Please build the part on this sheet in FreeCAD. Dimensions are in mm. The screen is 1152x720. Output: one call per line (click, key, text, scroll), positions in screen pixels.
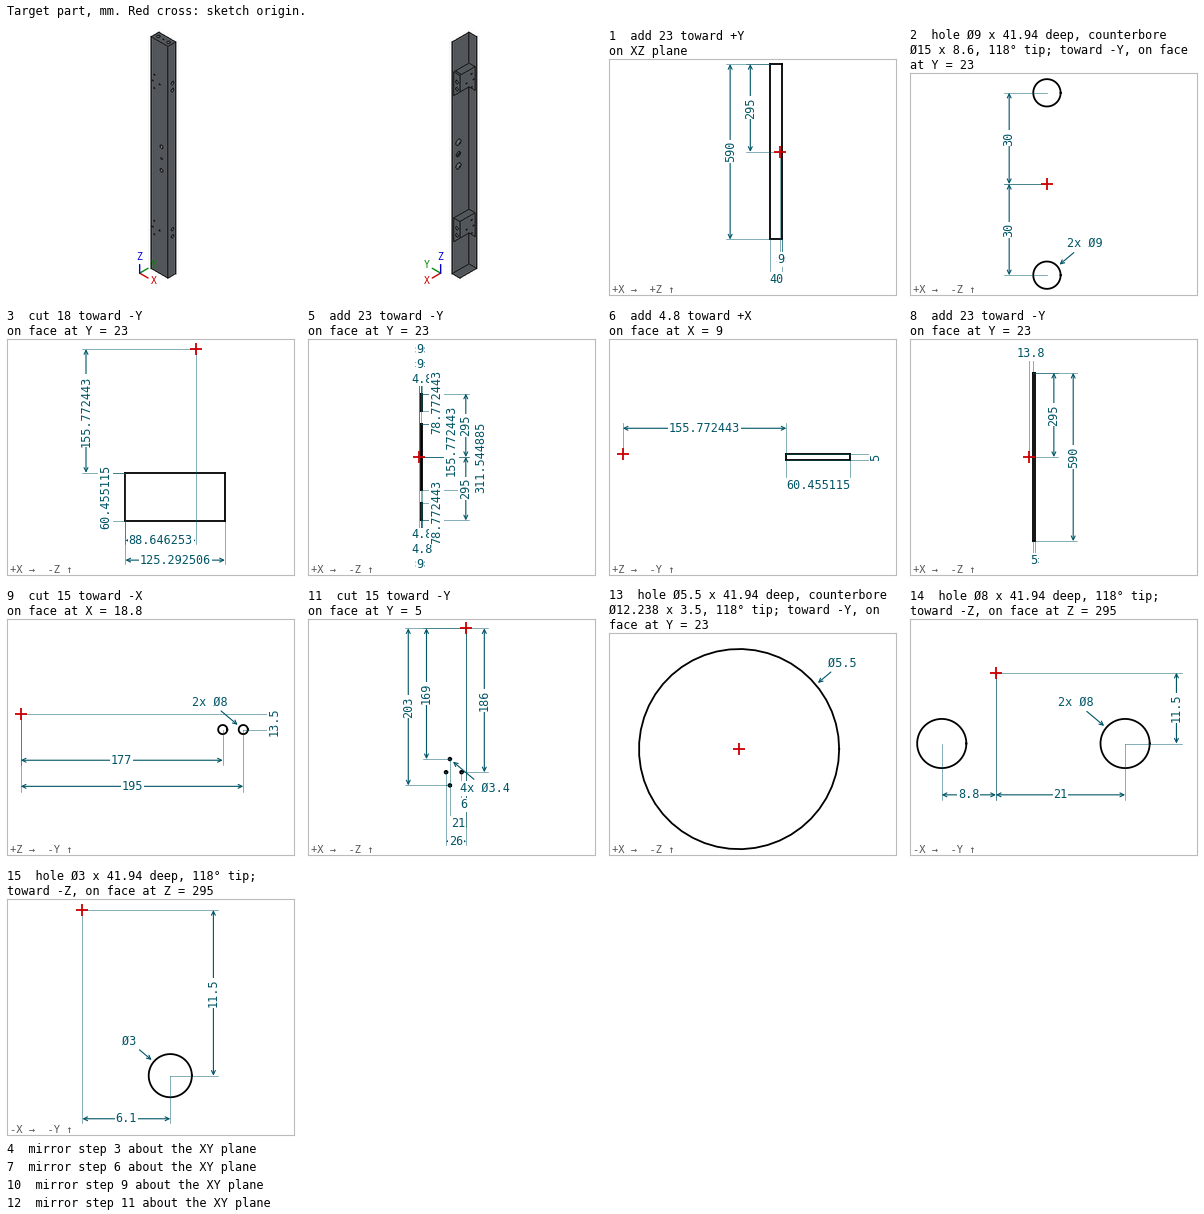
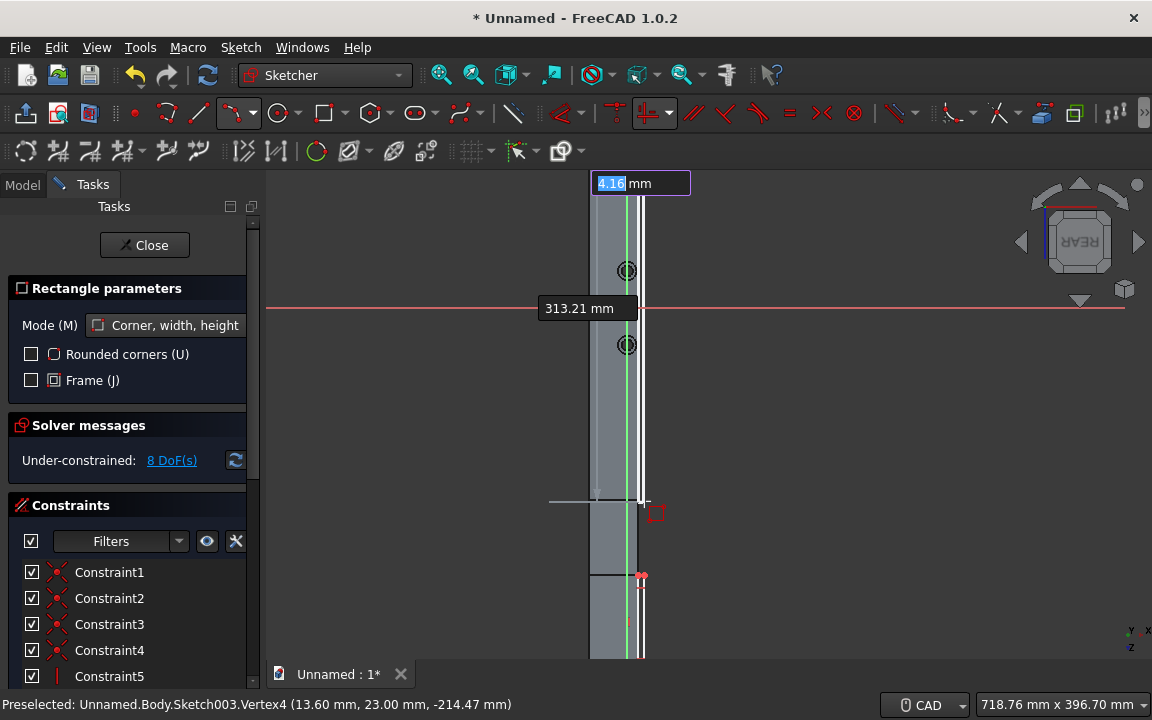
click(644, 500)
key(Escape)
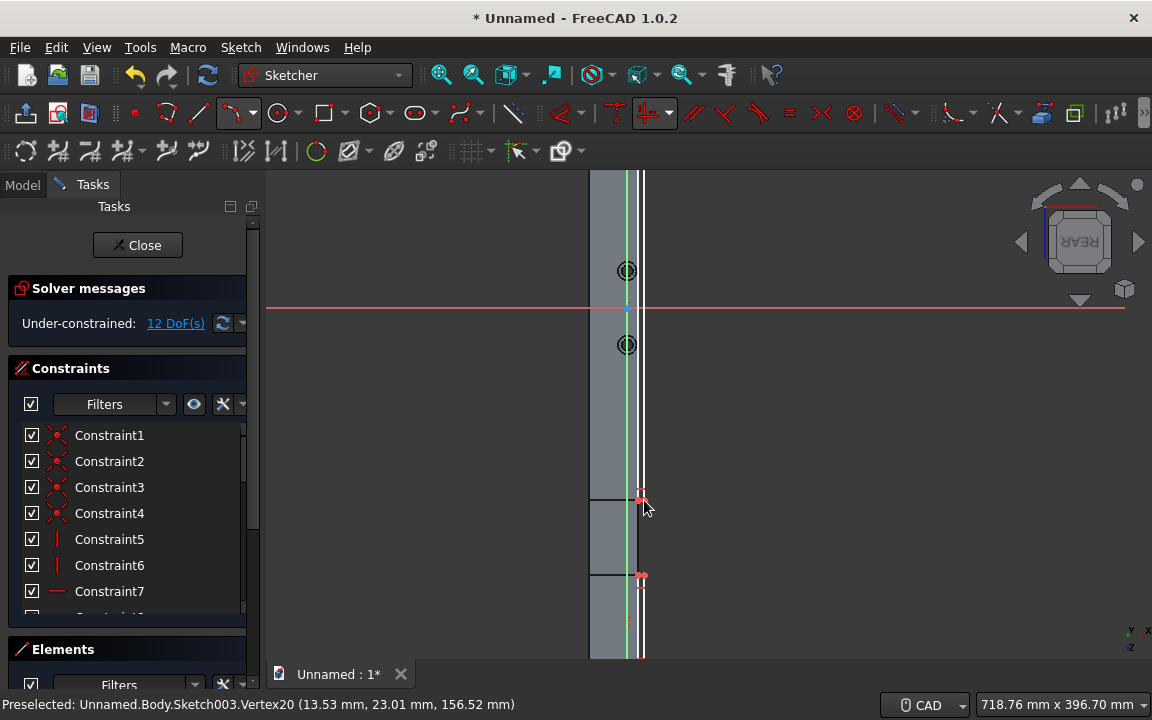
click(560, 114)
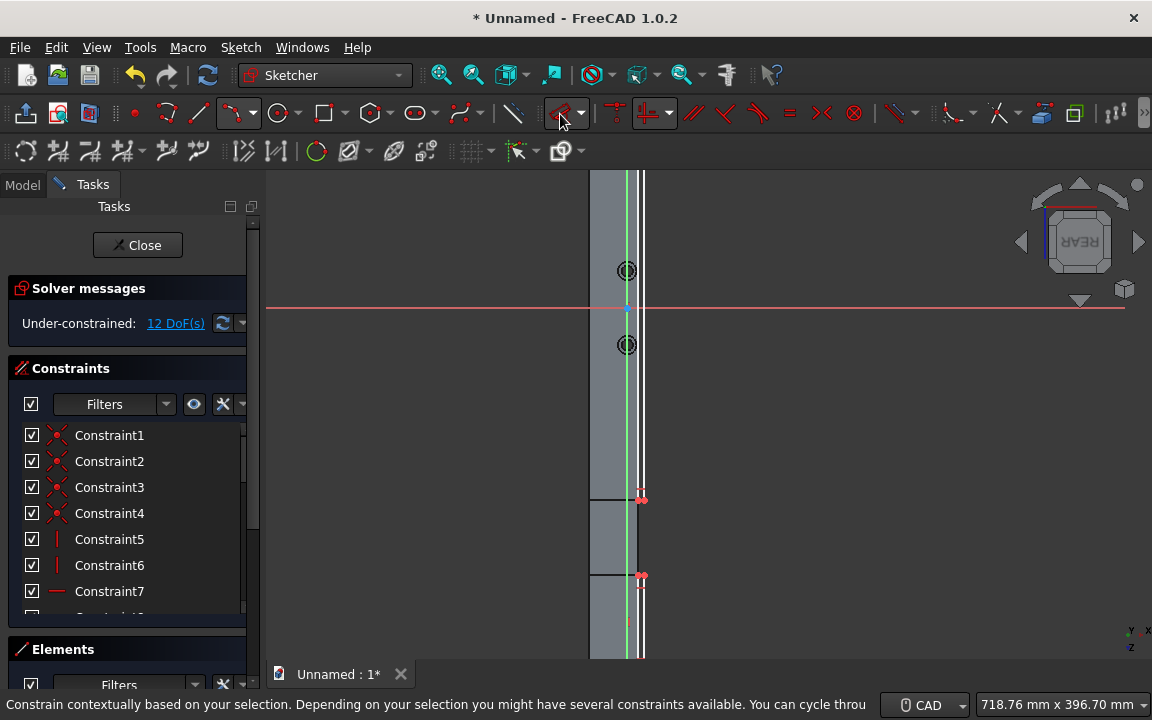
scroll(638, 575, up, 7)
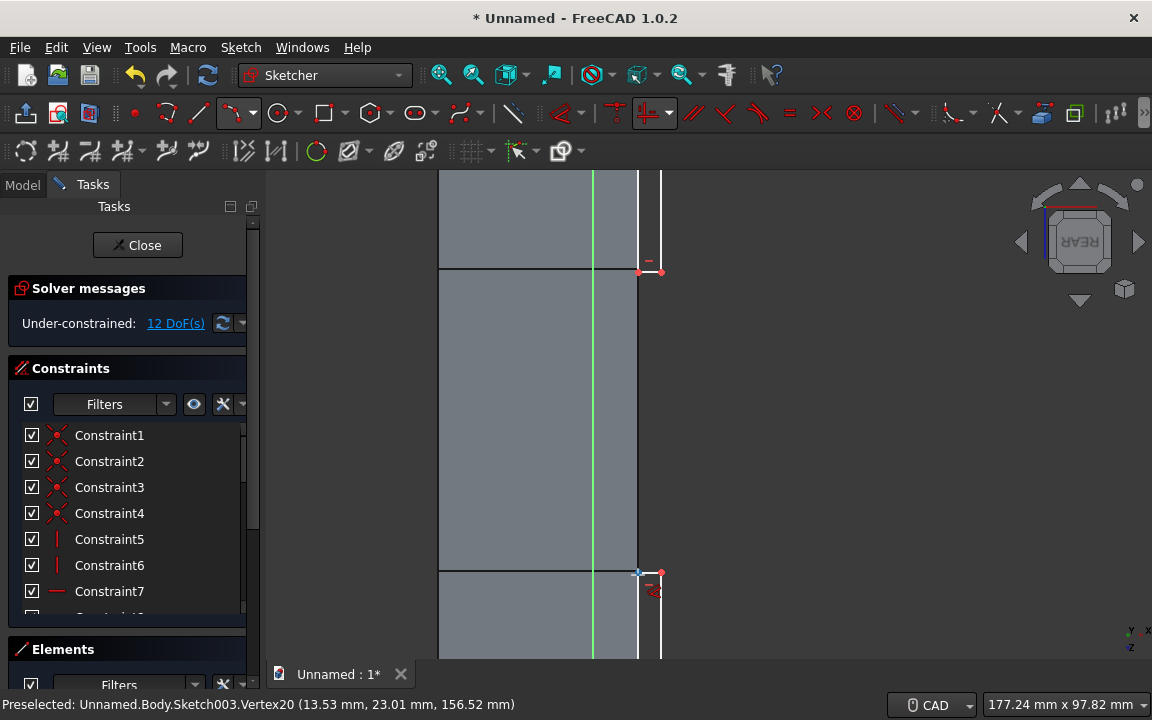
click(638, 573)
click(616, 607)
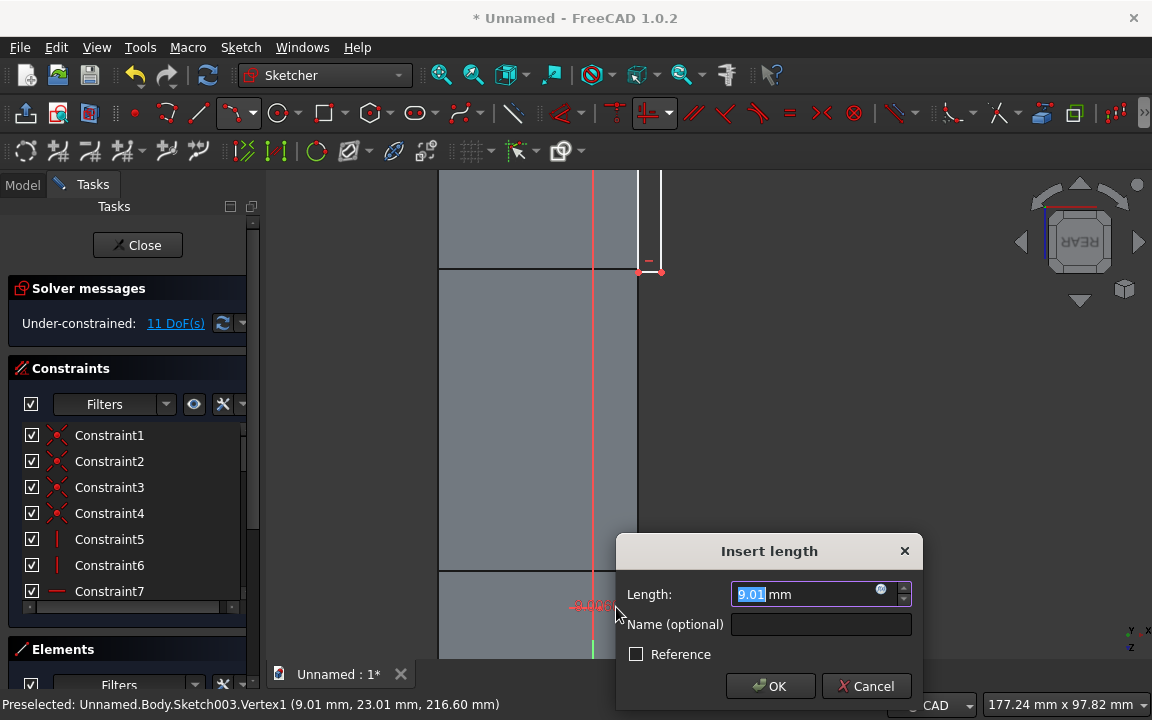
text(9)
key(Return)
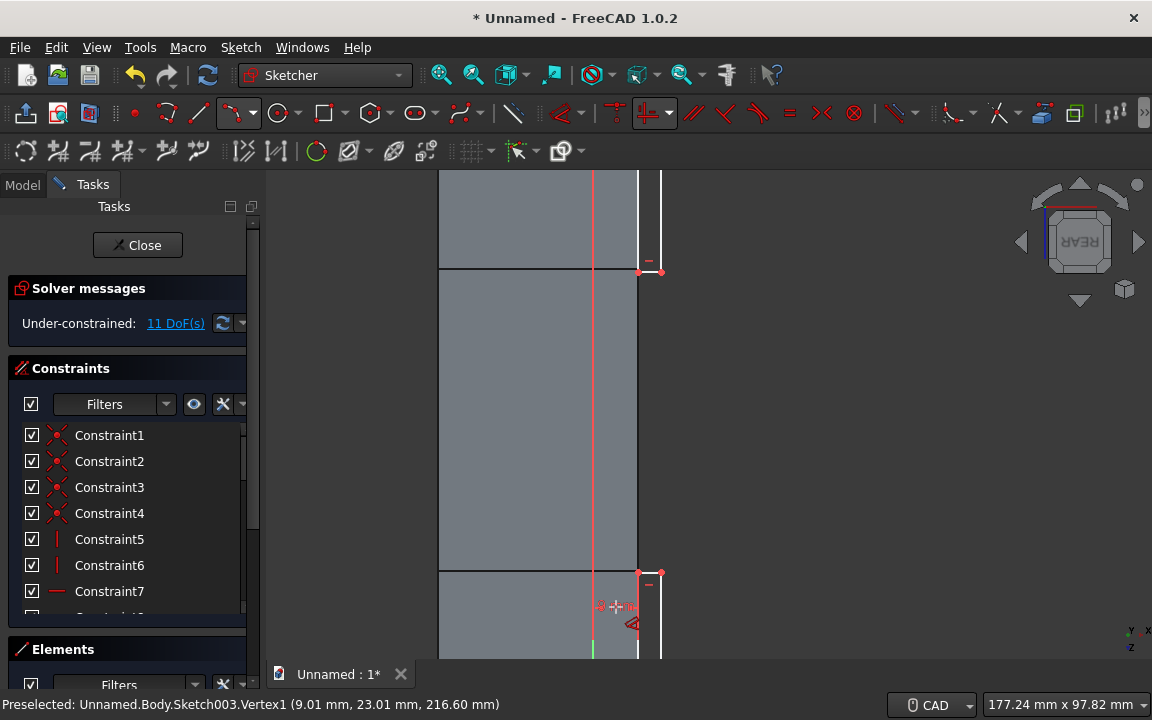
scroll(642, 530, down, 11)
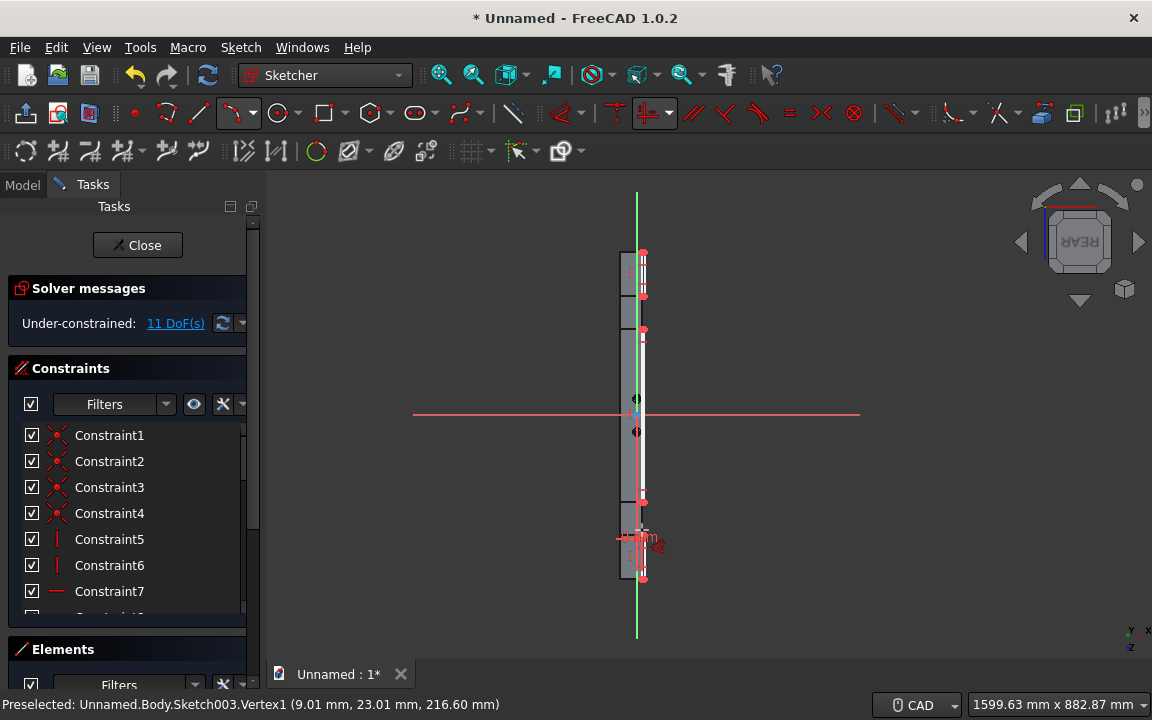
scroll(642, 252, up, 11)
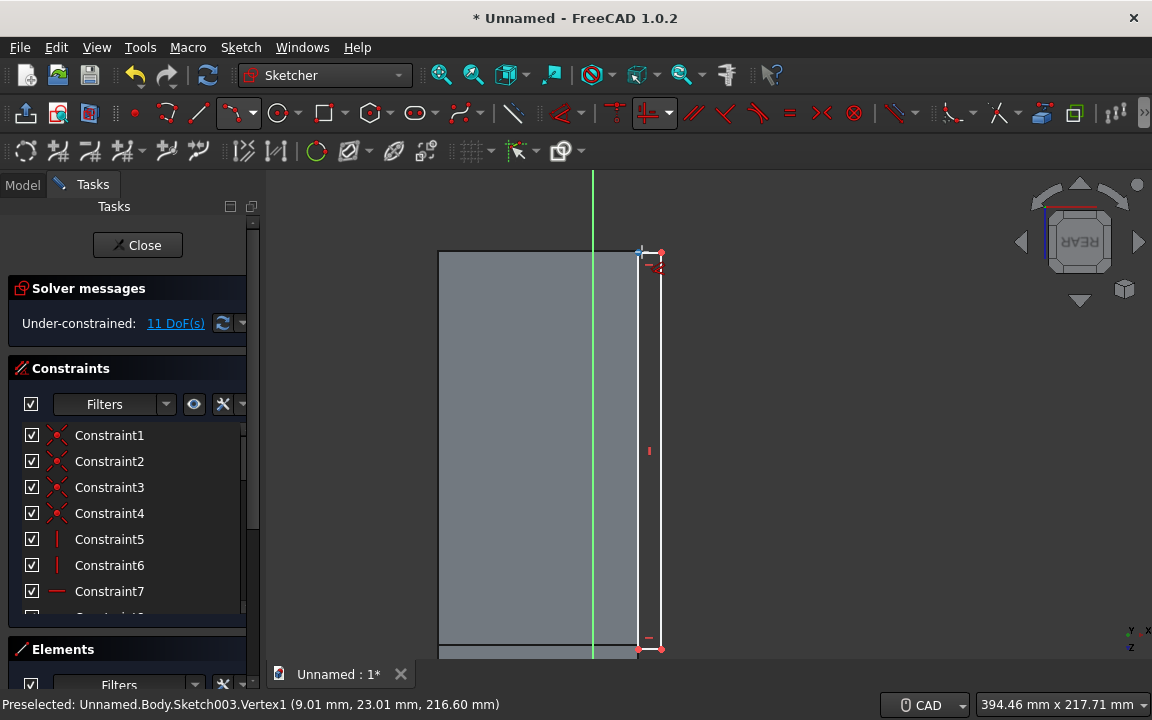
click(638, 253)
click(616, 219)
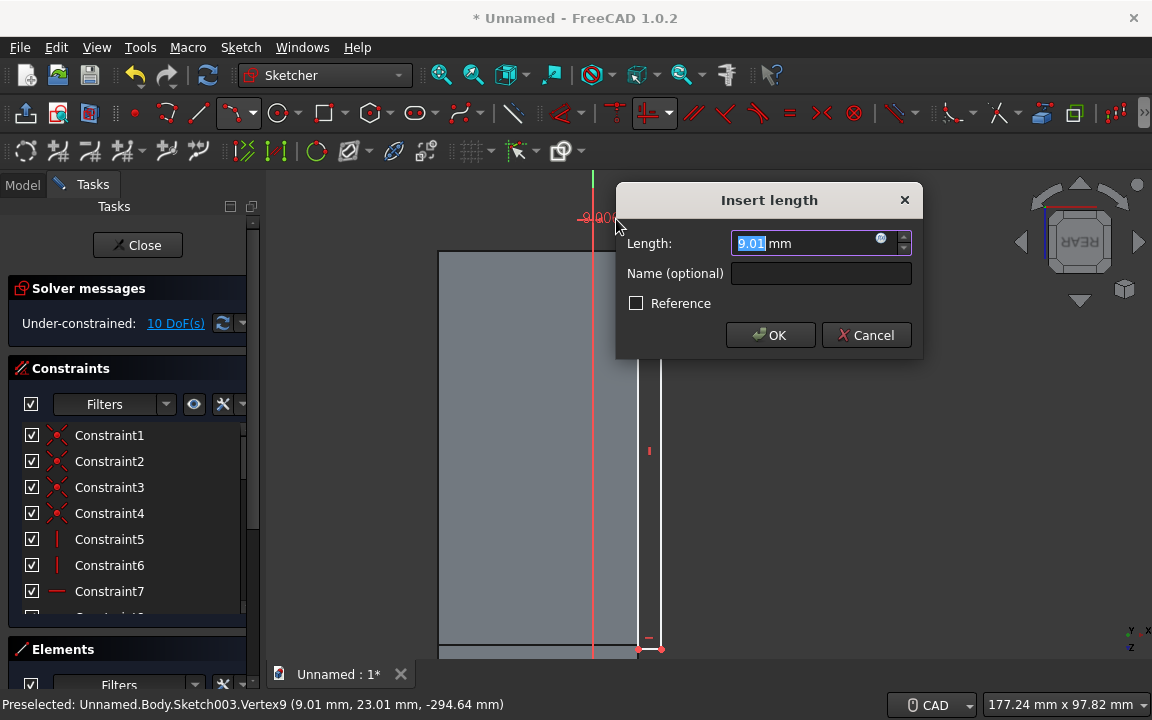
text(9)
key(Return)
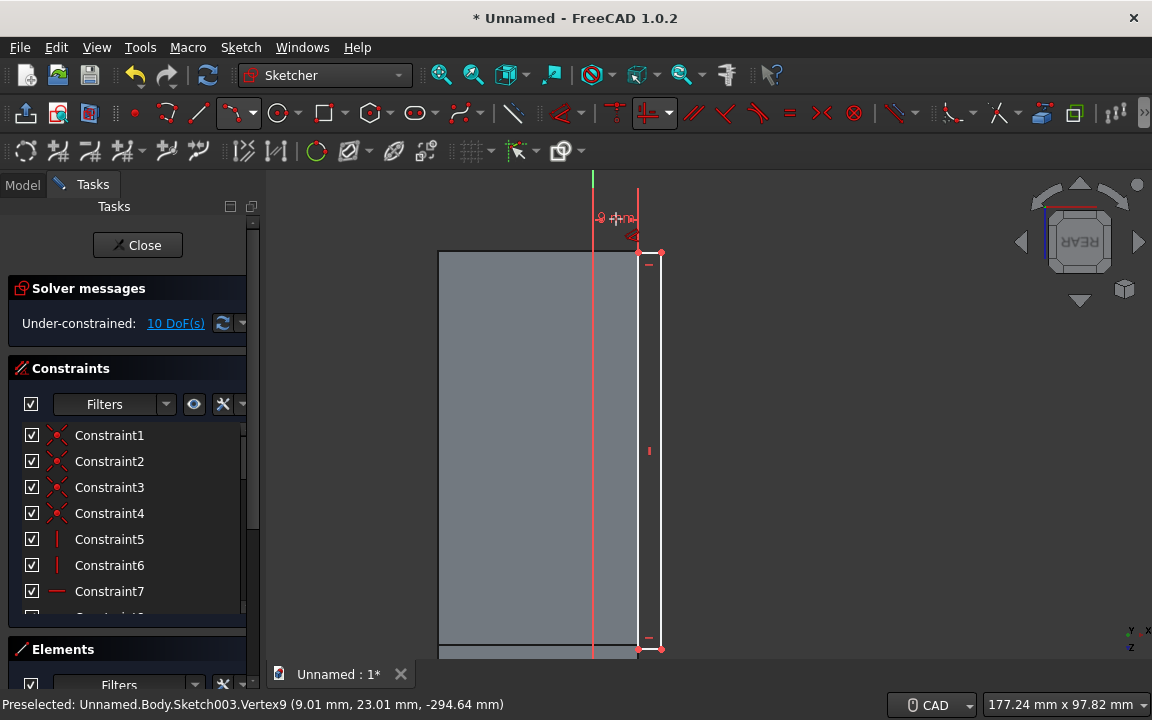
scroll(642, 251, down, 11)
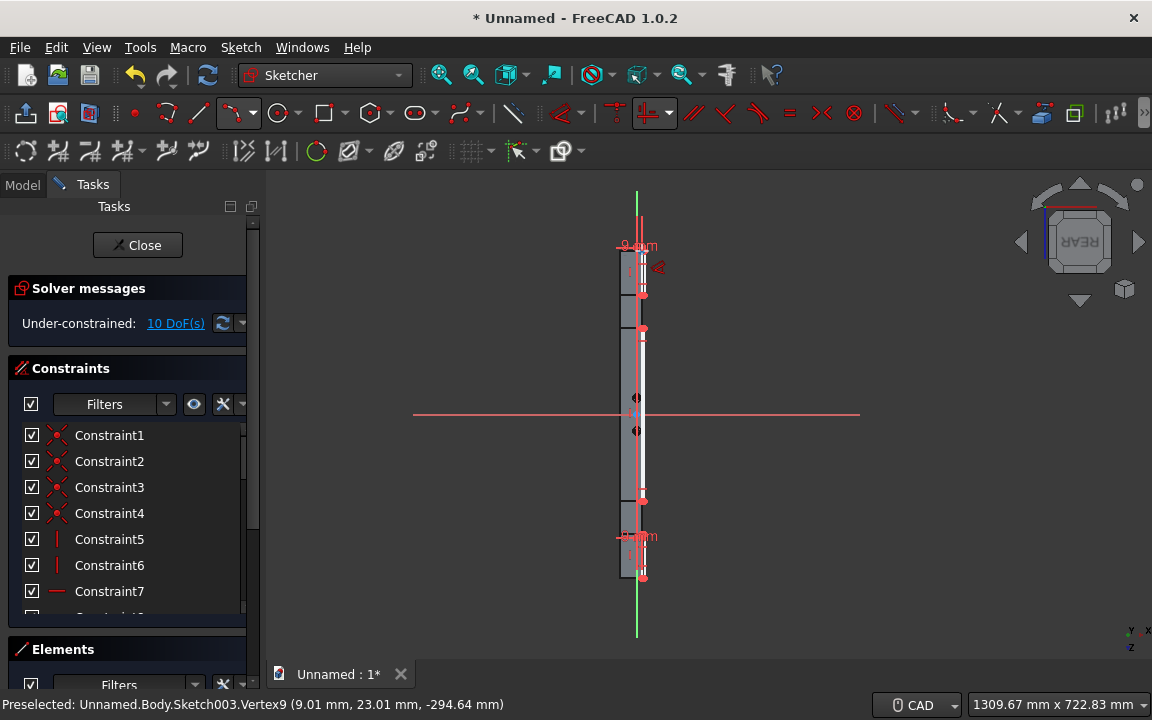
scroll(642, 328, up, 11)